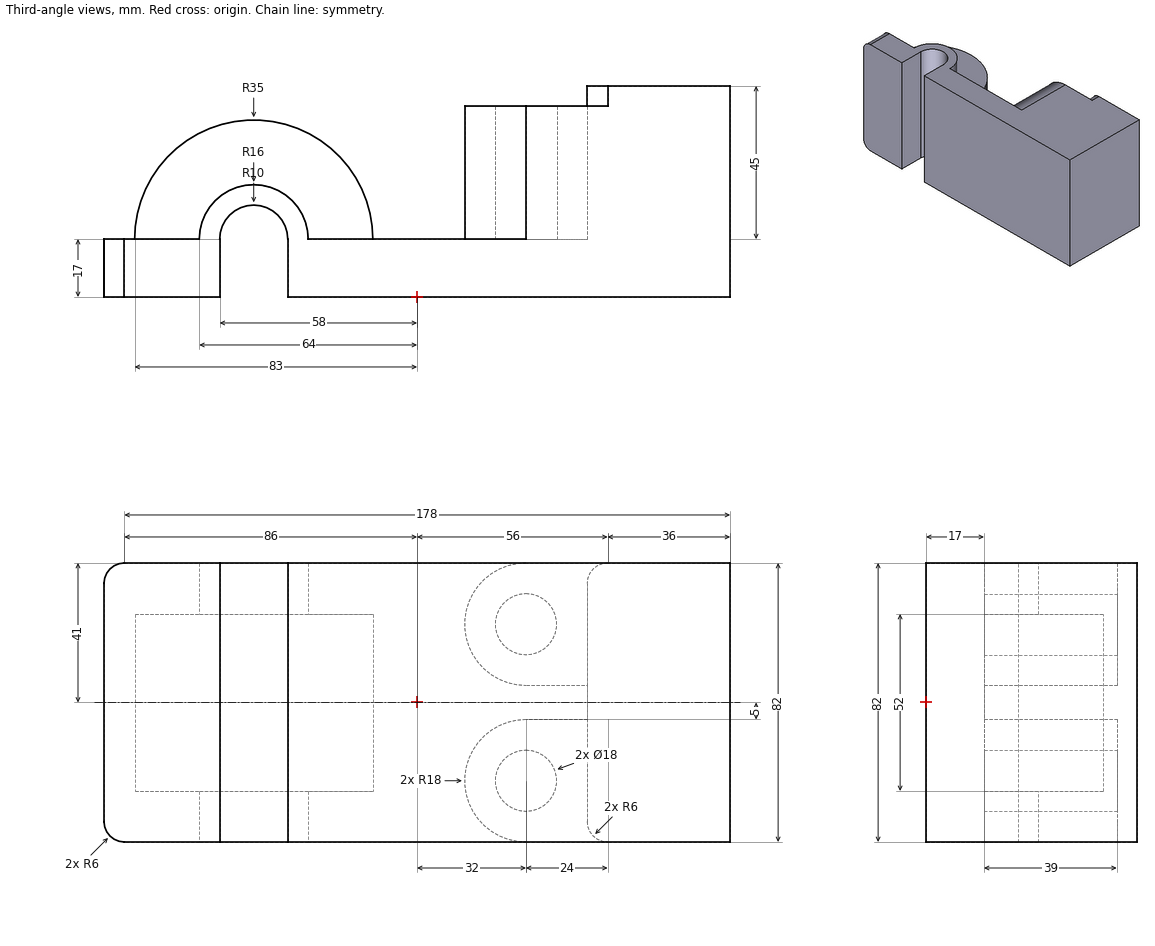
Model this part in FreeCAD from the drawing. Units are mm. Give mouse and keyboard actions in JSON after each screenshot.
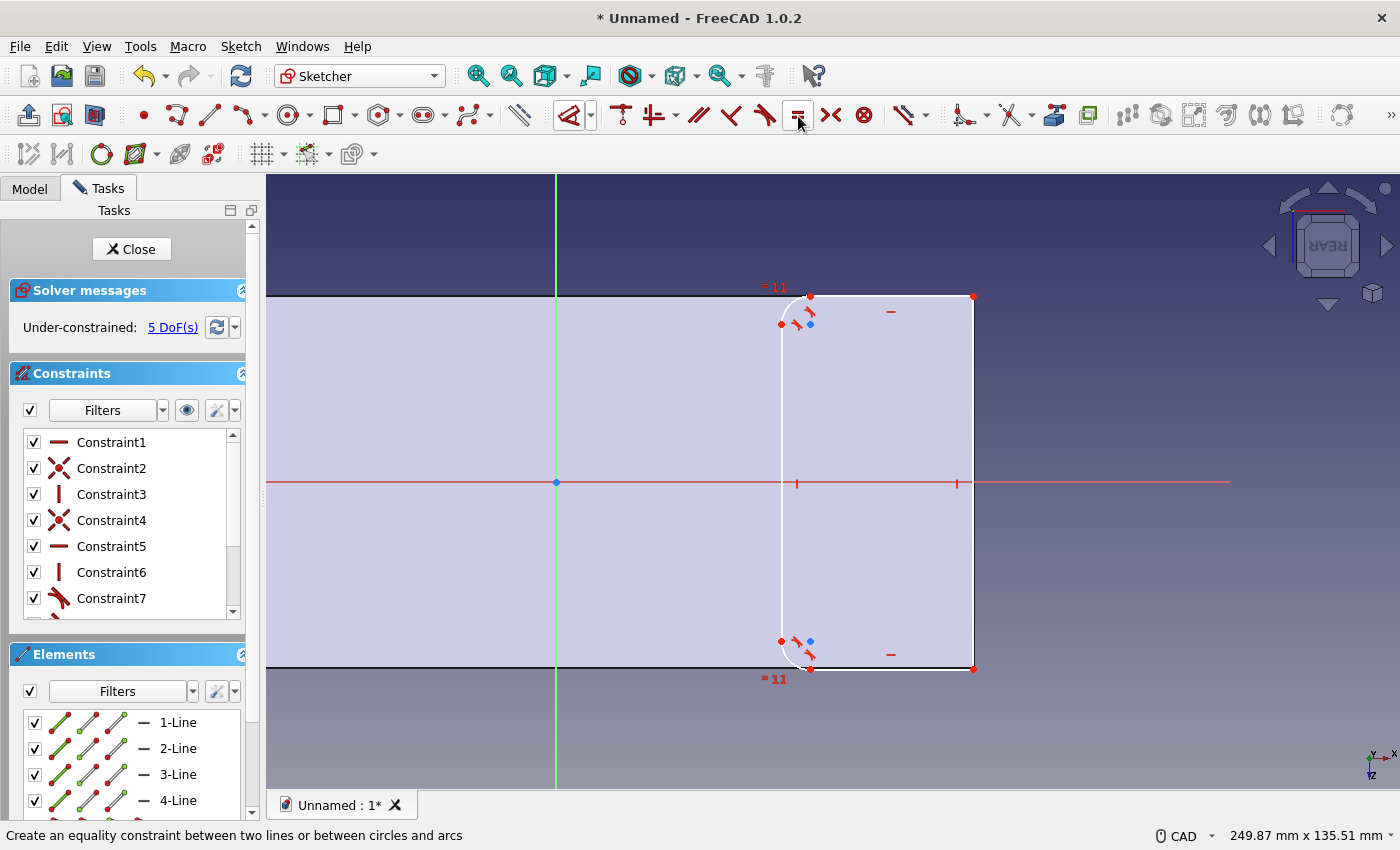
{"action": "scroll", "coordinate": [797, 299], "scroll_direction": "up", "scroll_amount": 2}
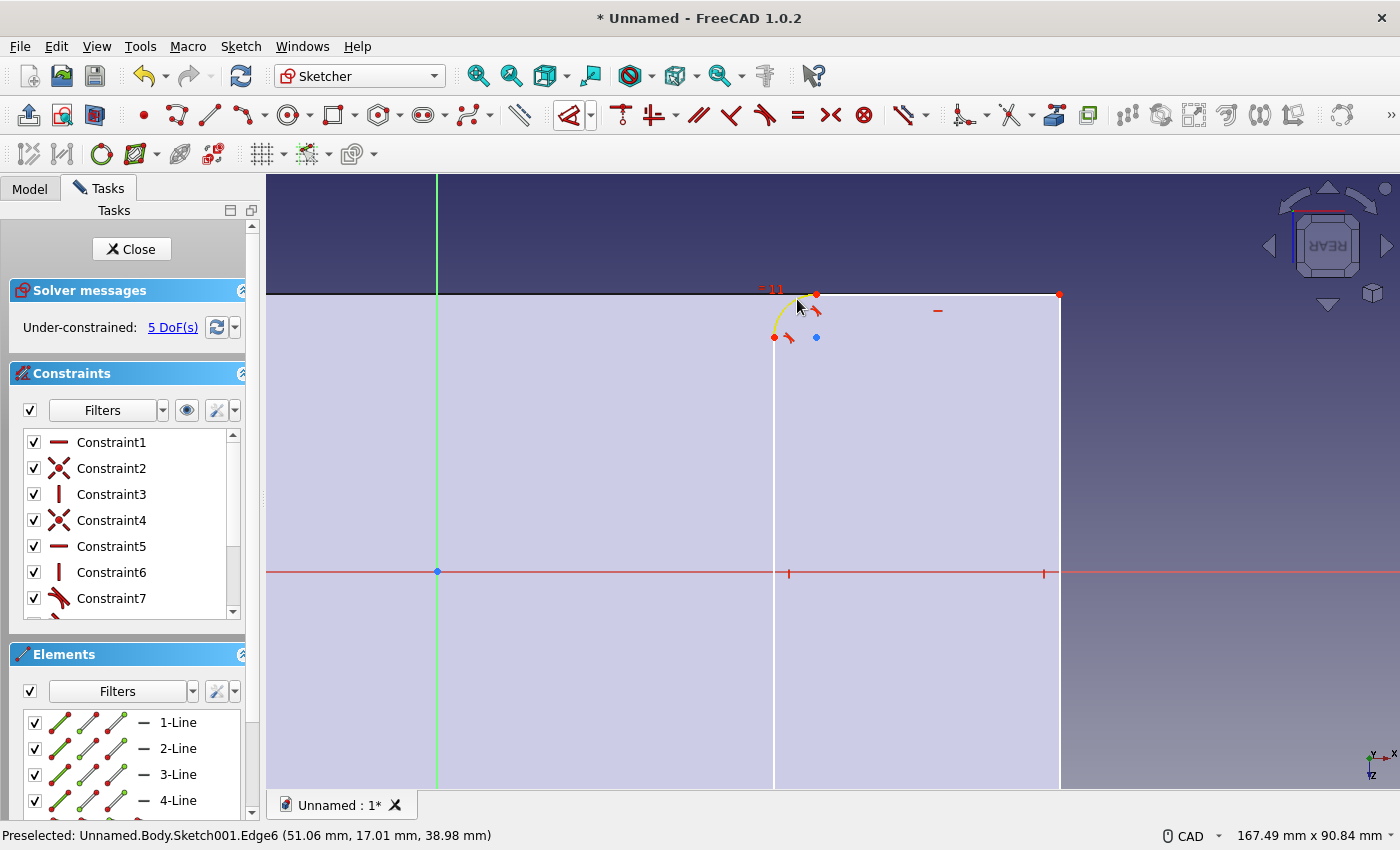
{"action": "left_click", "coordinate": [797, 299]}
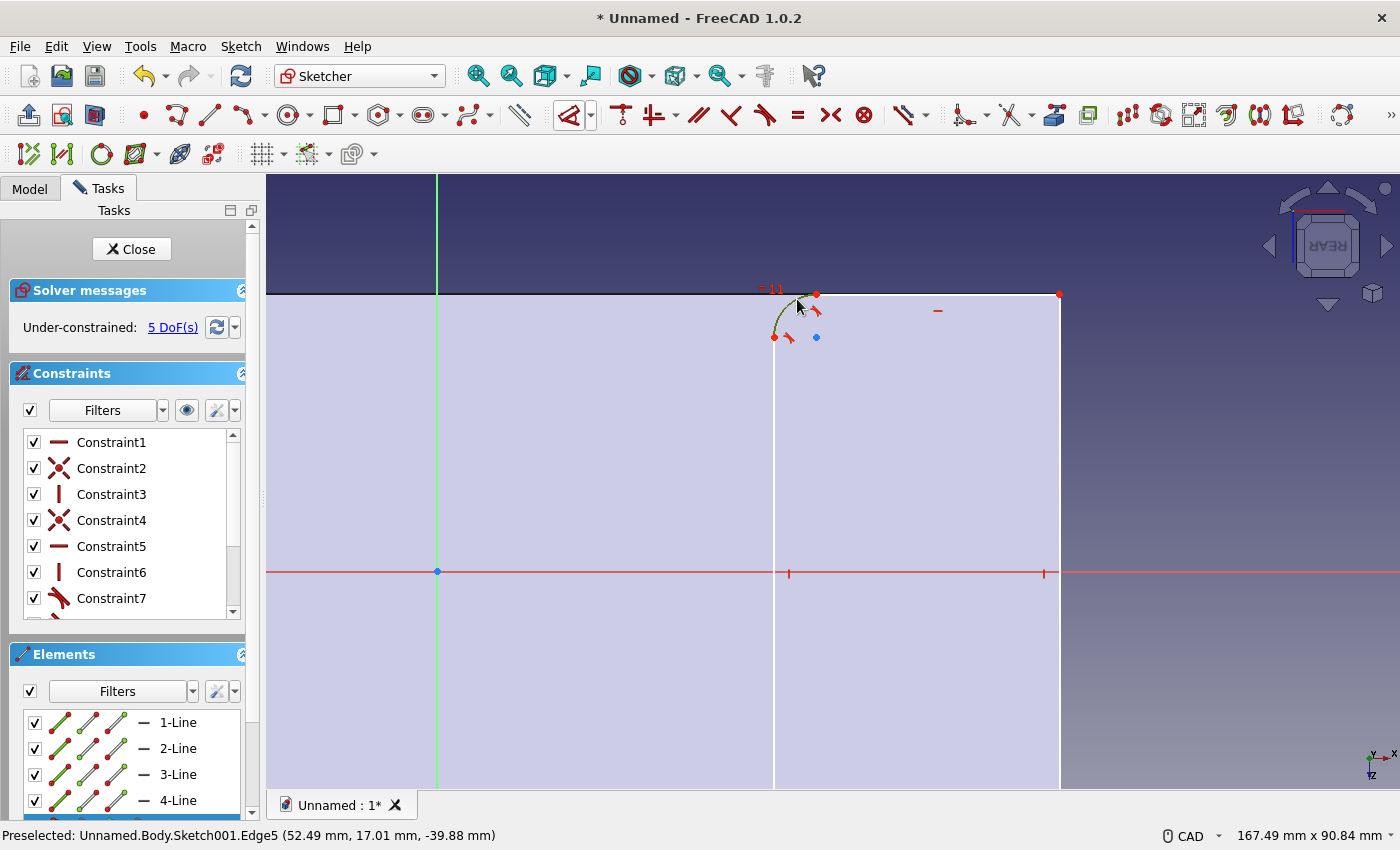
{"action": "key", "text": "k r"}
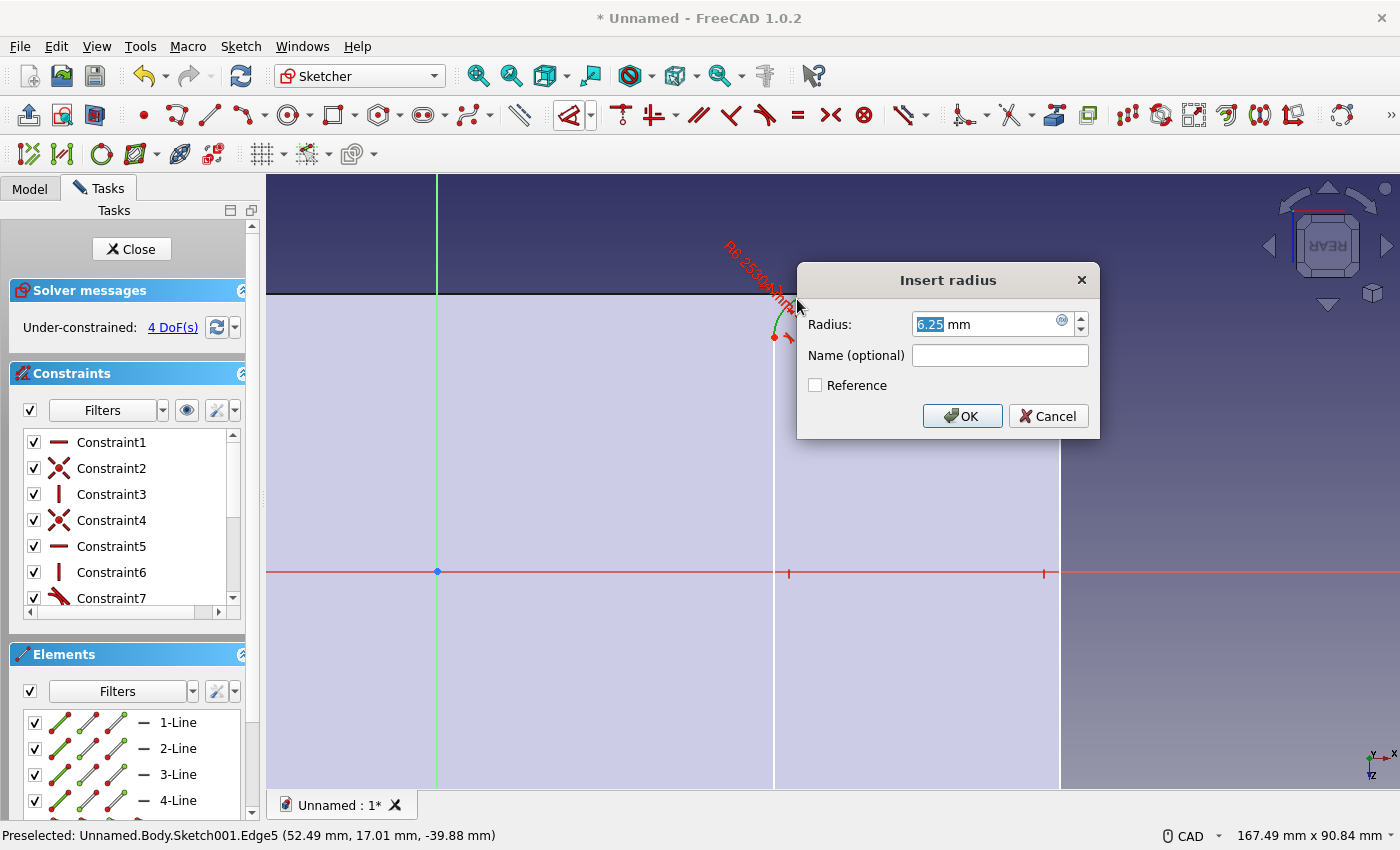
{"action": "type", "text": "6"}
{"action": "key", "text": "Return"}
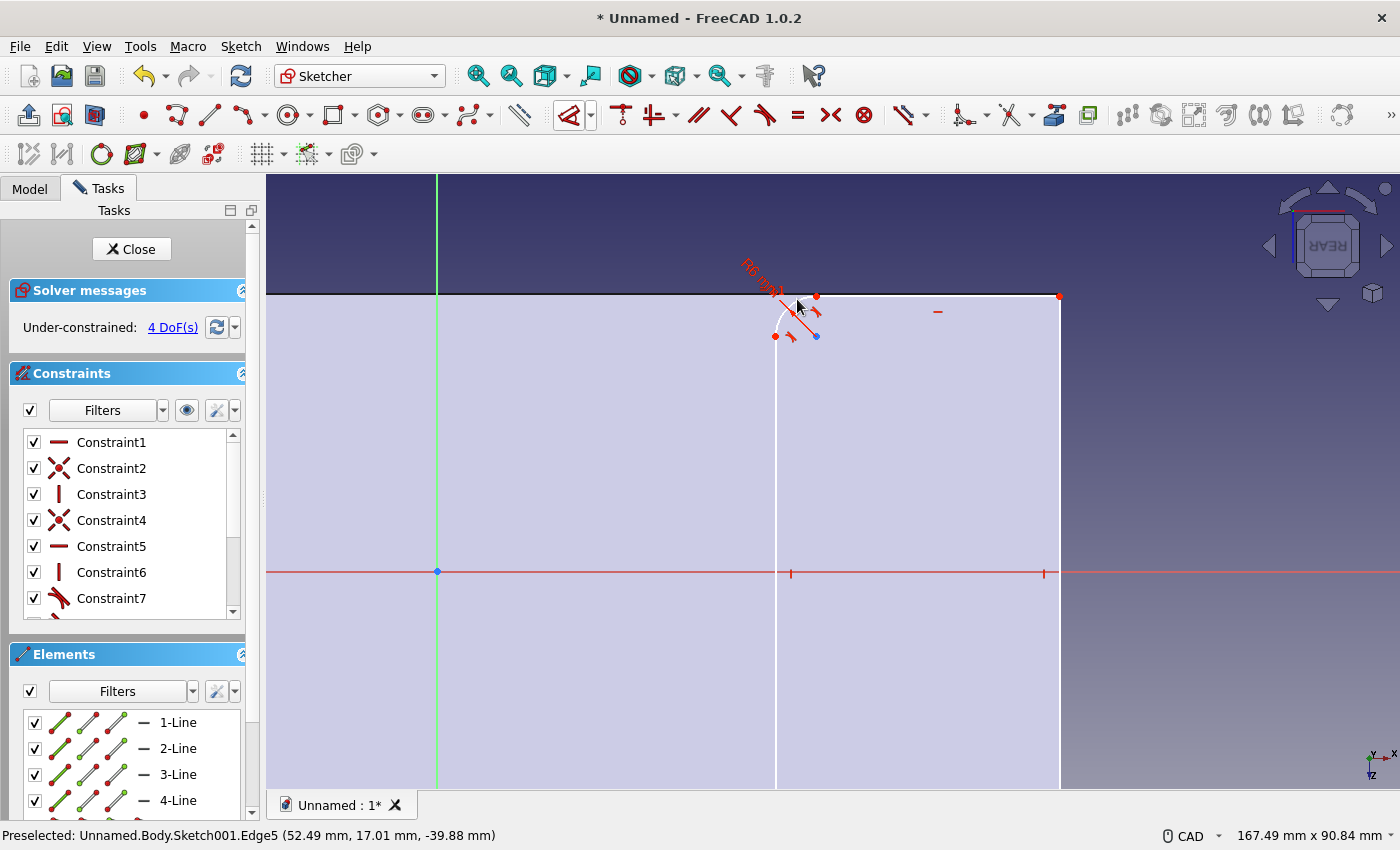
{"action": "scroll", "coordinate": [797, 298], "scroll_direction": "down", "scroll_amount": 2}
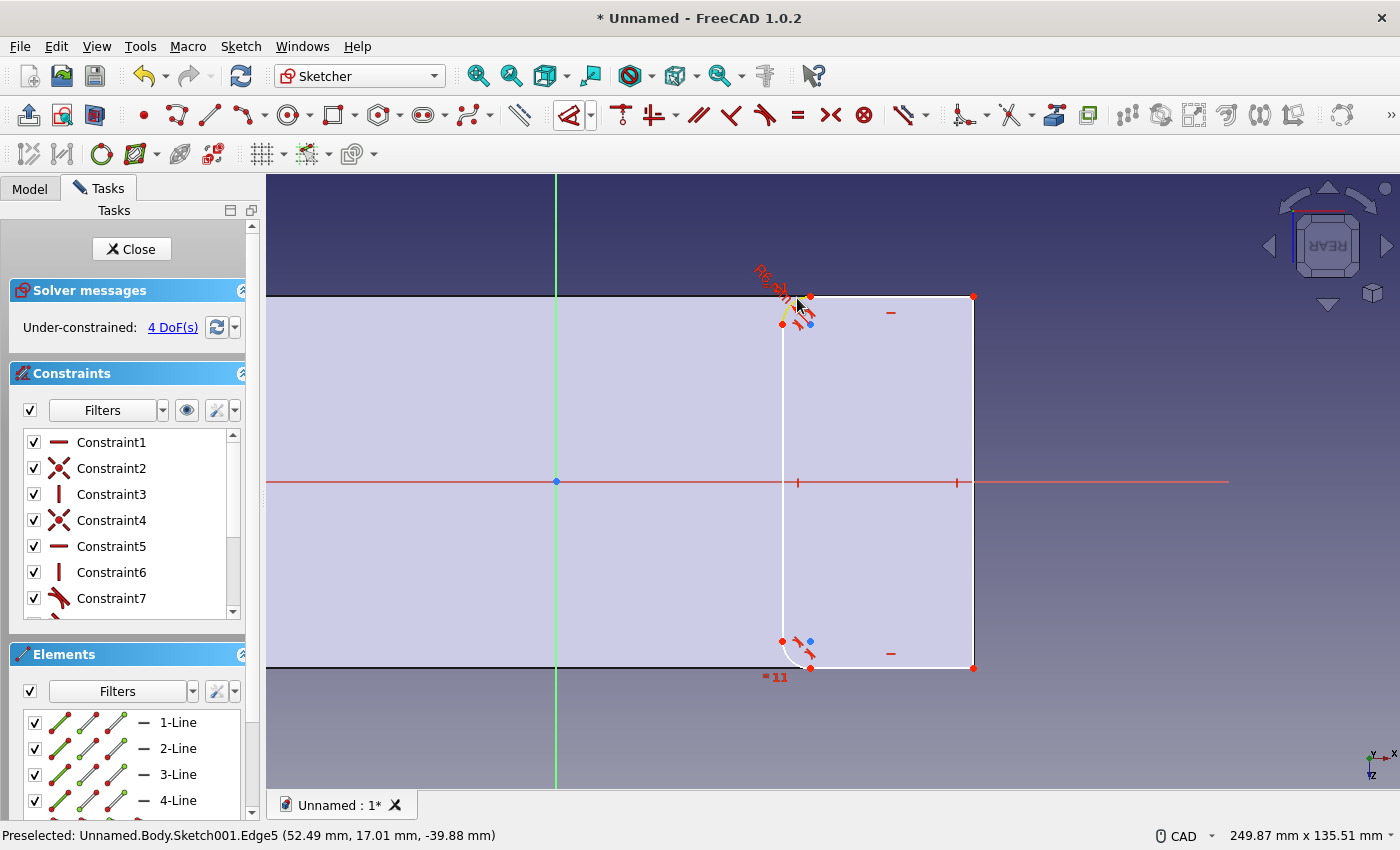
{"action": "left_click", "coordinate": [859, 668]}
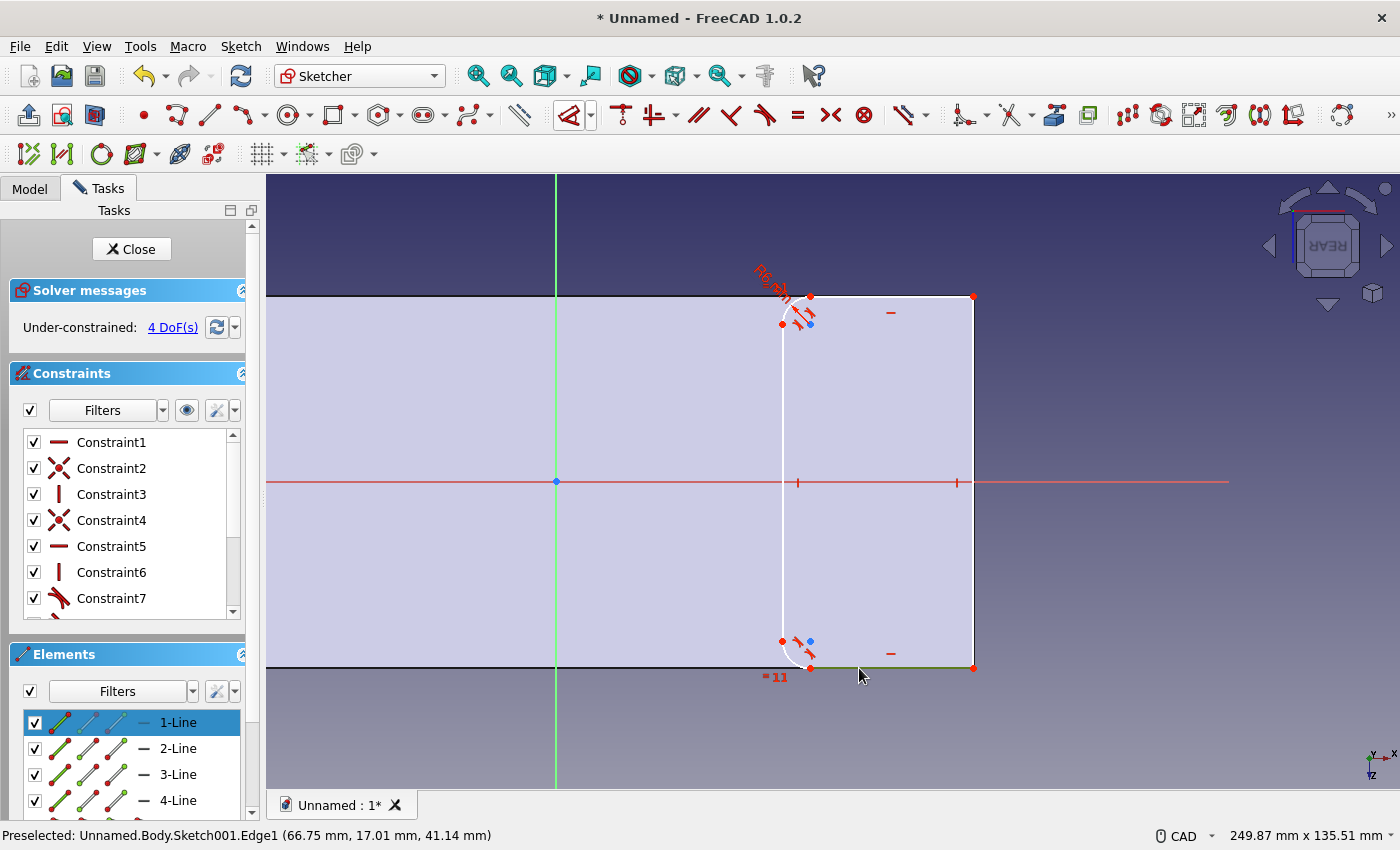
{"action": "left_click", "coordinate": [590, 116]}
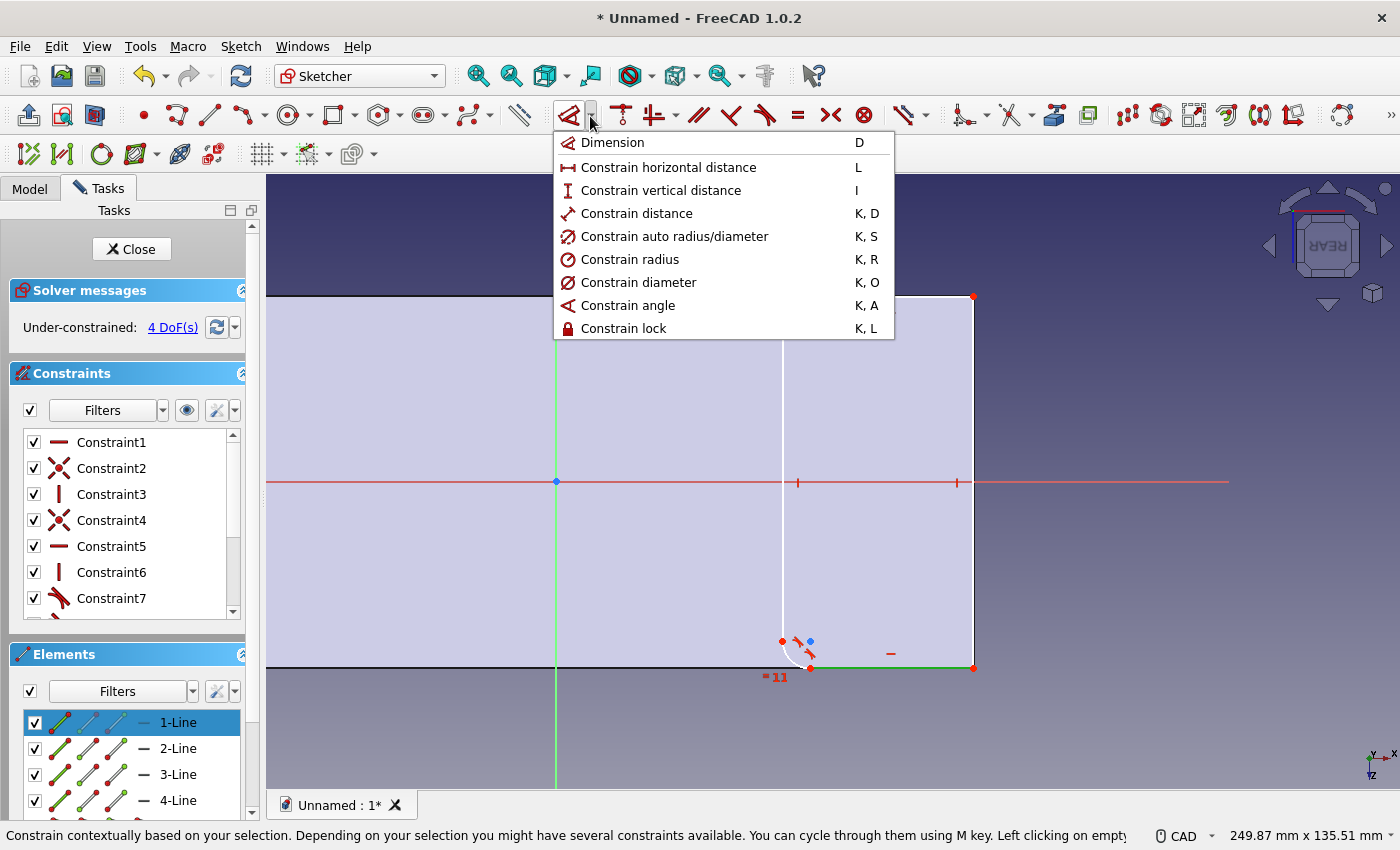
{"action": "left_click", "coordinate": [724, 168]}